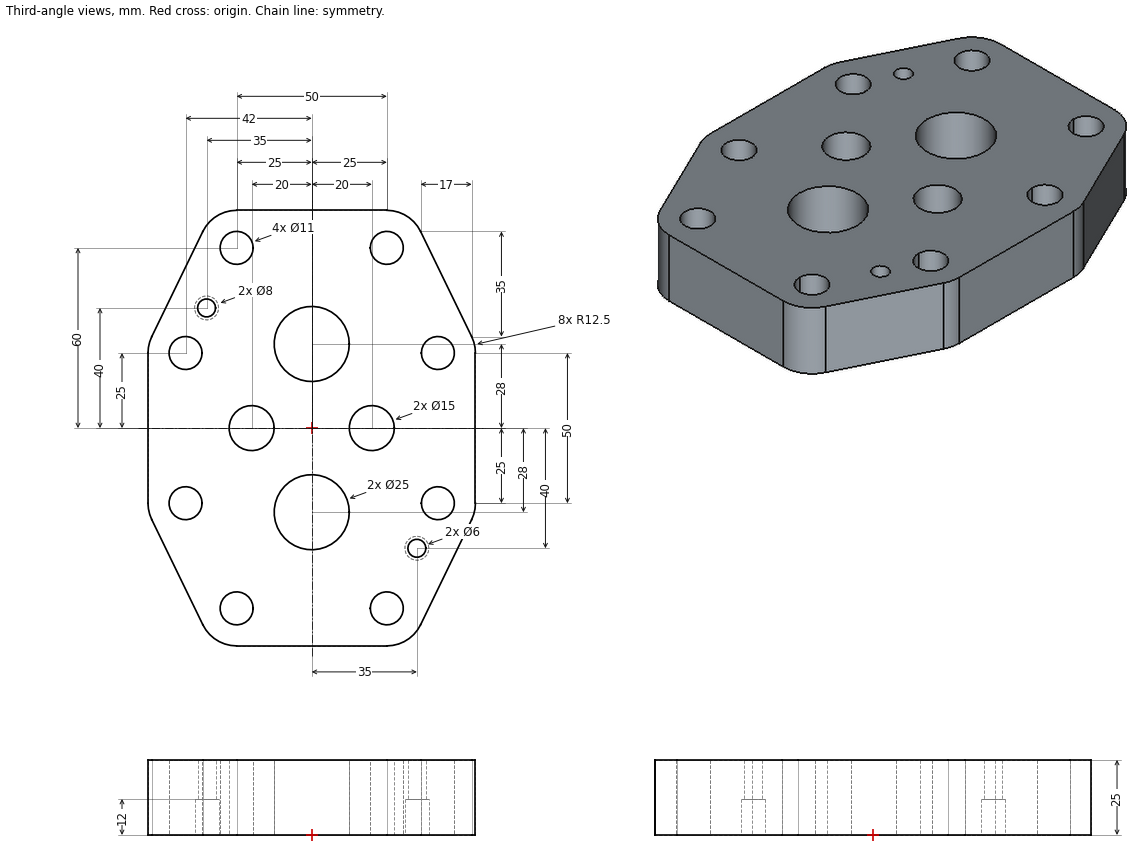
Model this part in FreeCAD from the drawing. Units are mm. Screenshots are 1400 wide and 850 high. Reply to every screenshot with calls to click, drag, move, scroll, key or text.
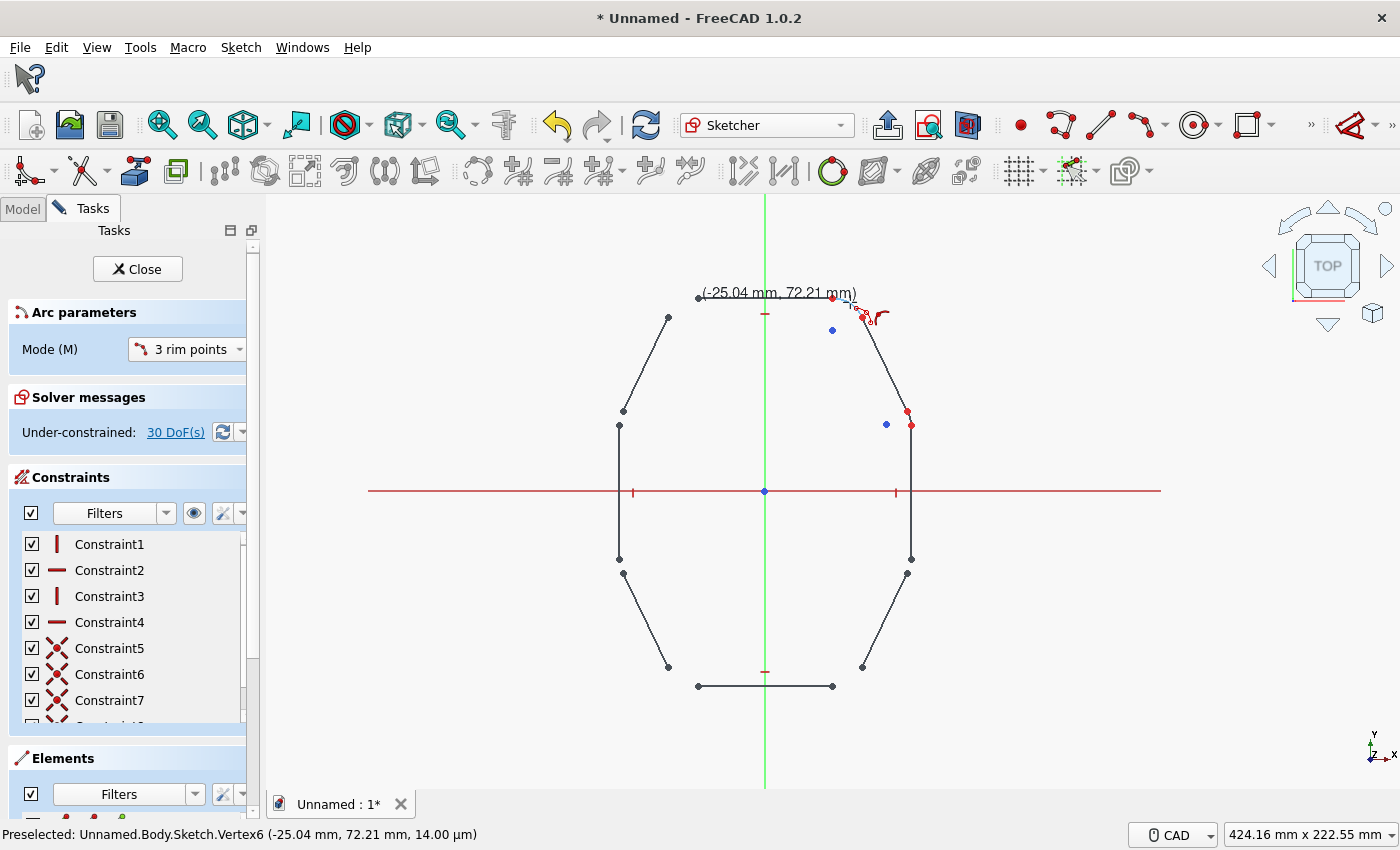
click(668, 317)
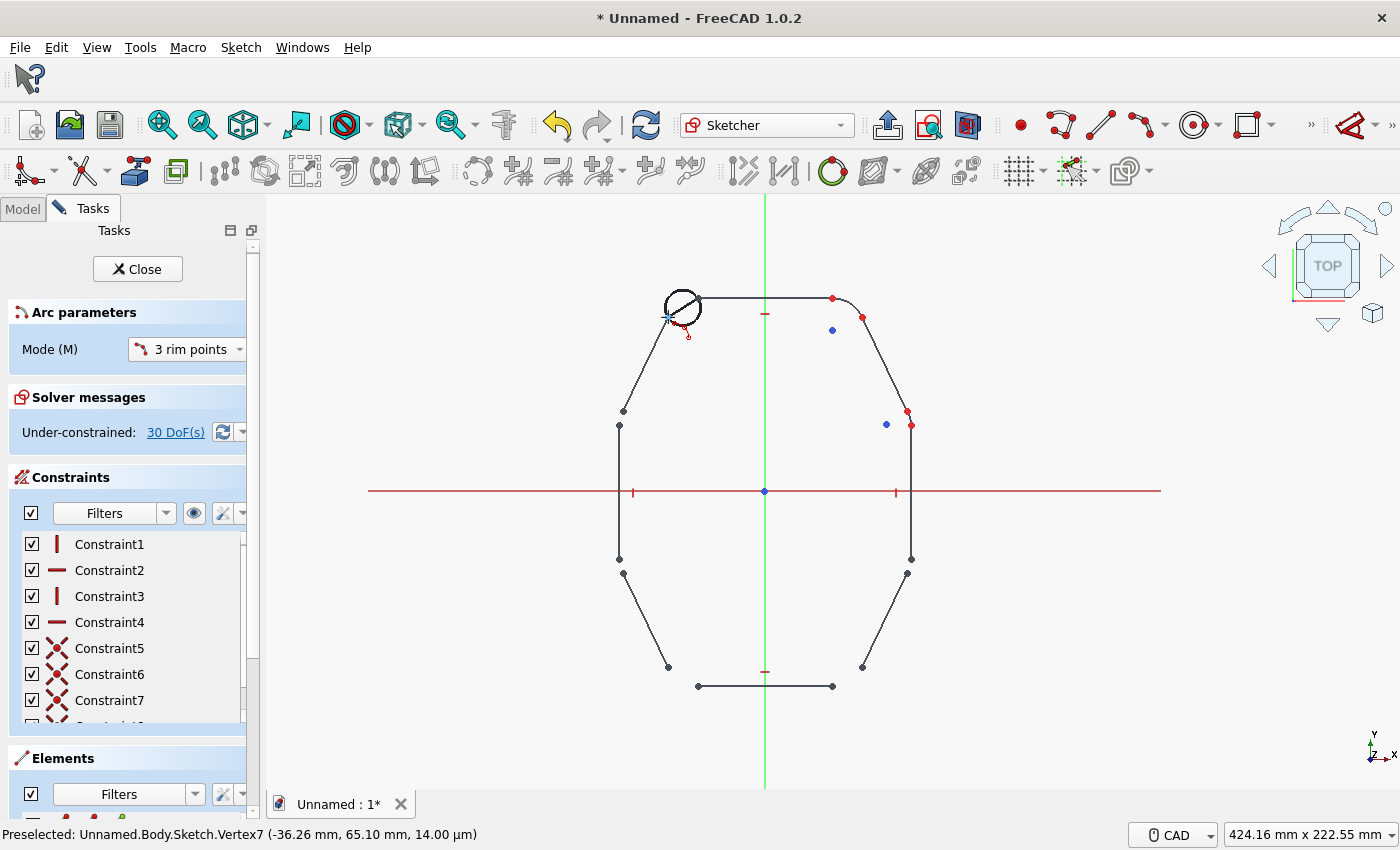
scroll(680, 303, up, 6)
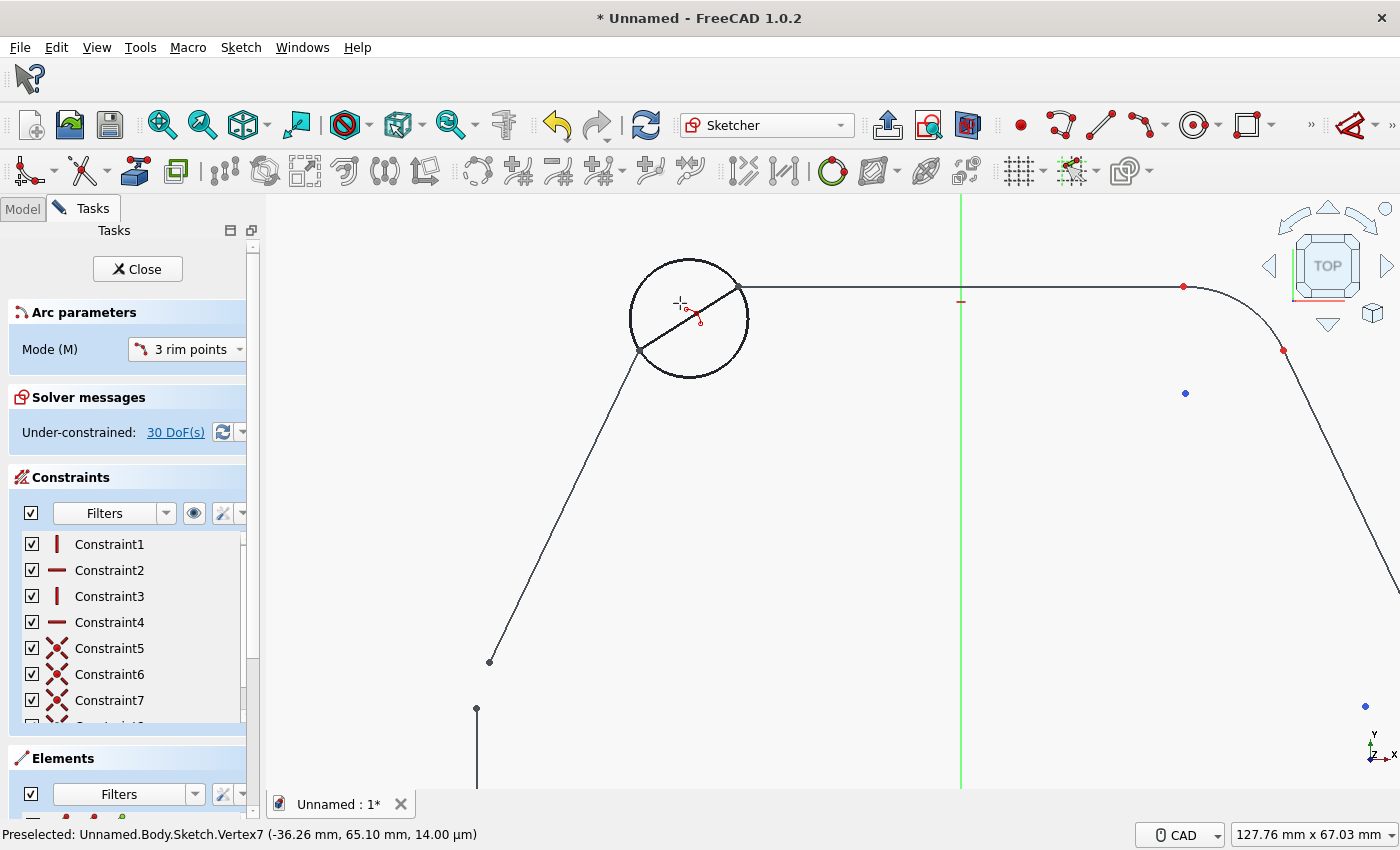
click(680, 301)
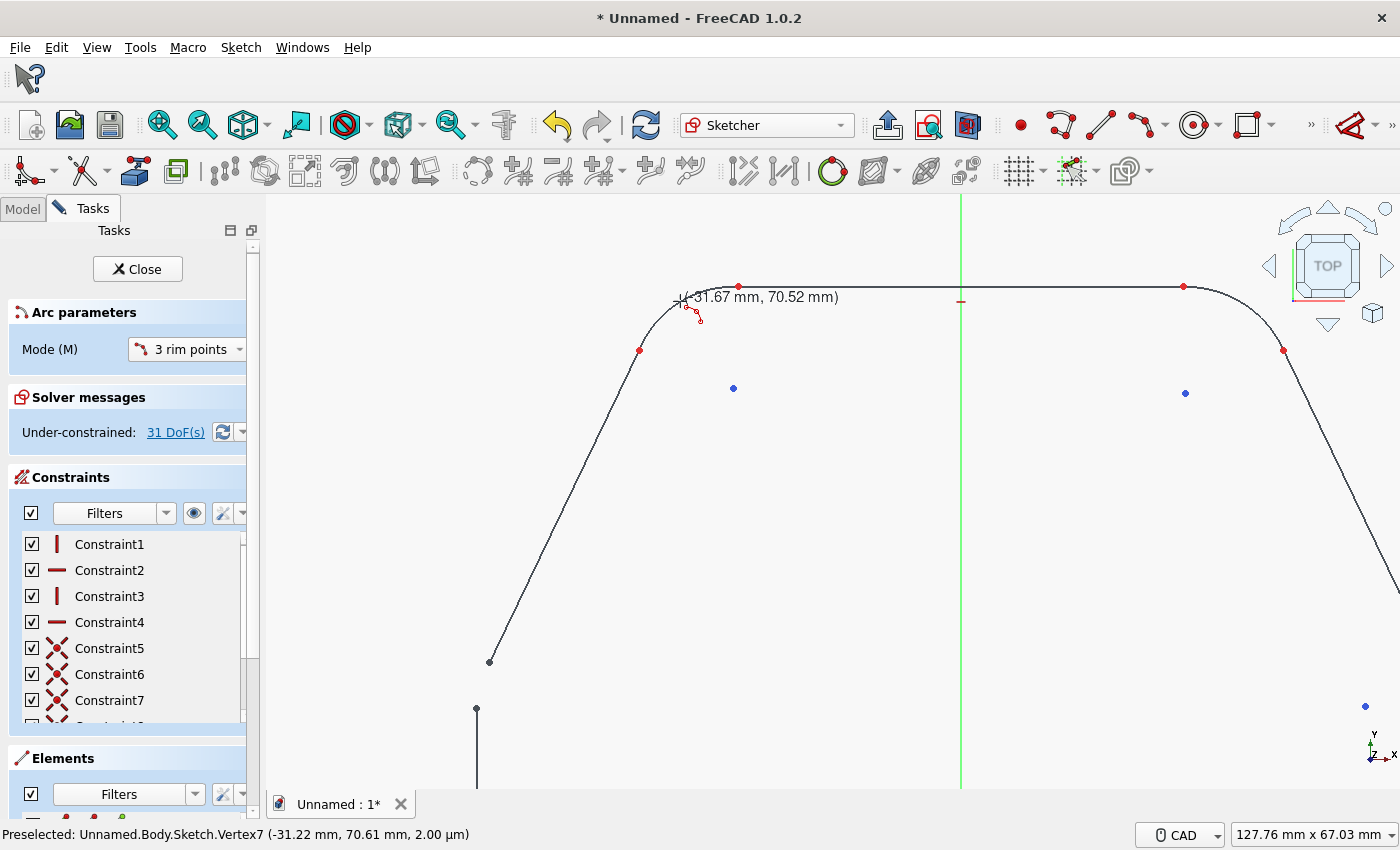
click(490, 662)
click(477, 709)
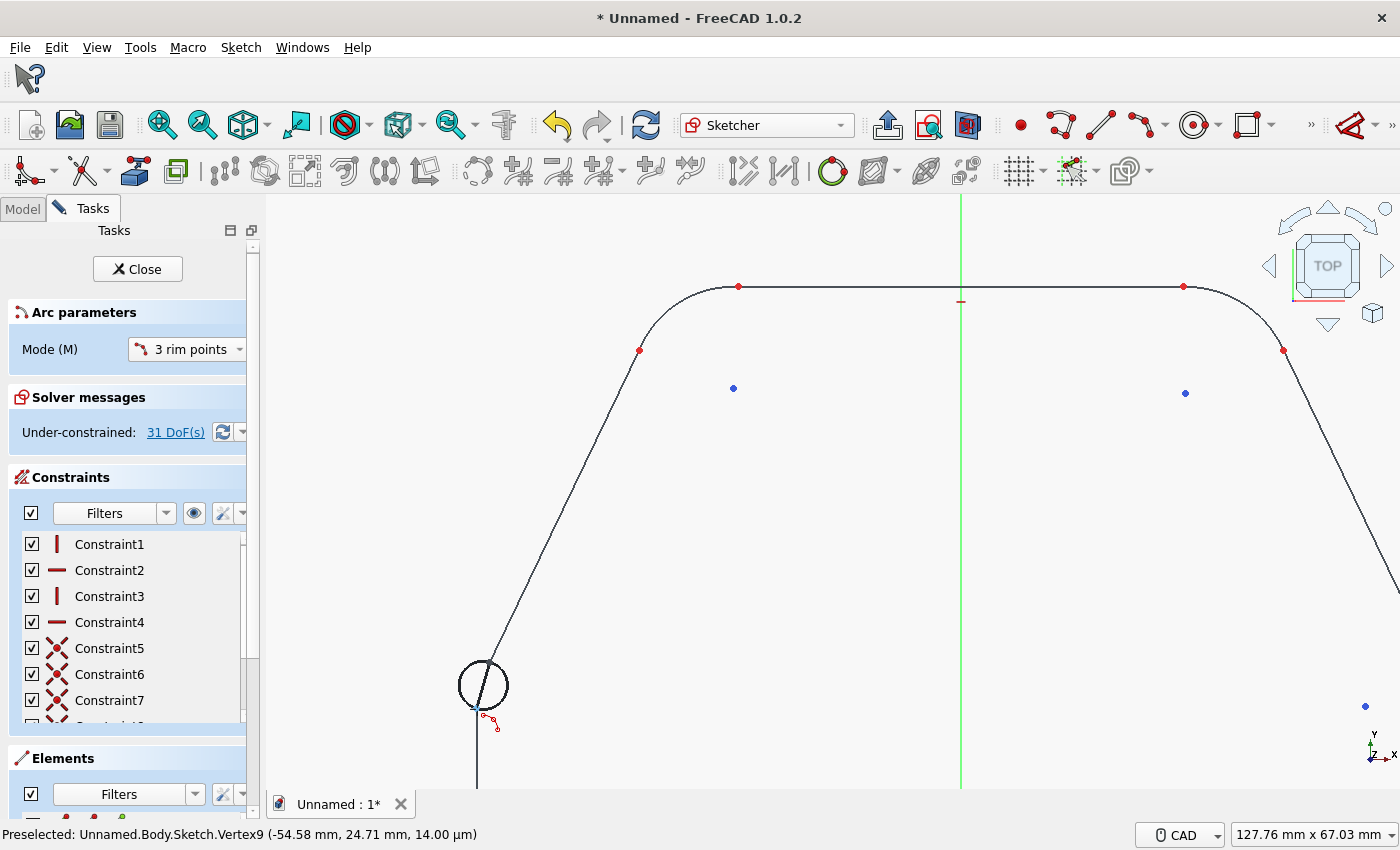
scroll(480, 681, up, 9)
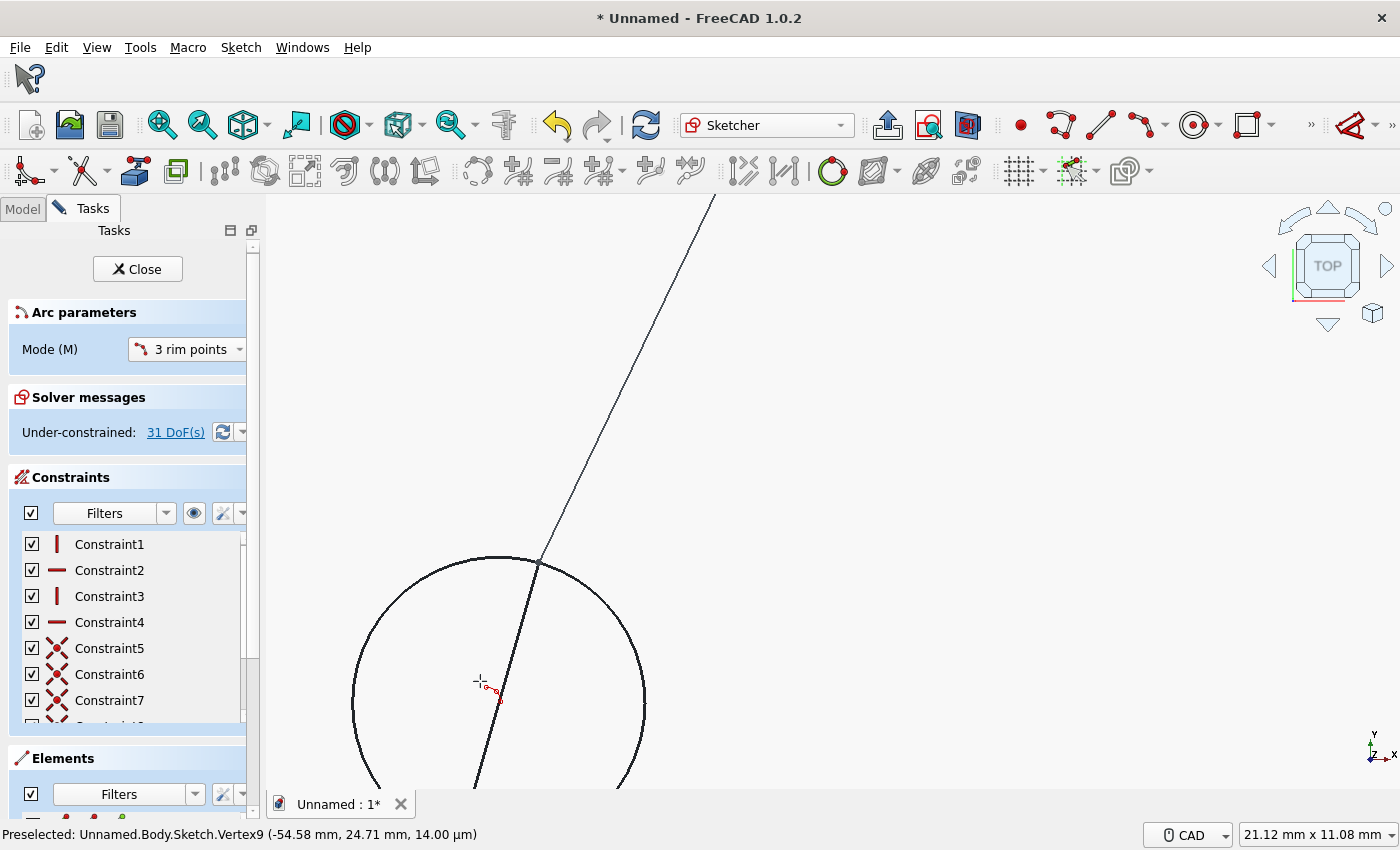
click(480, 678)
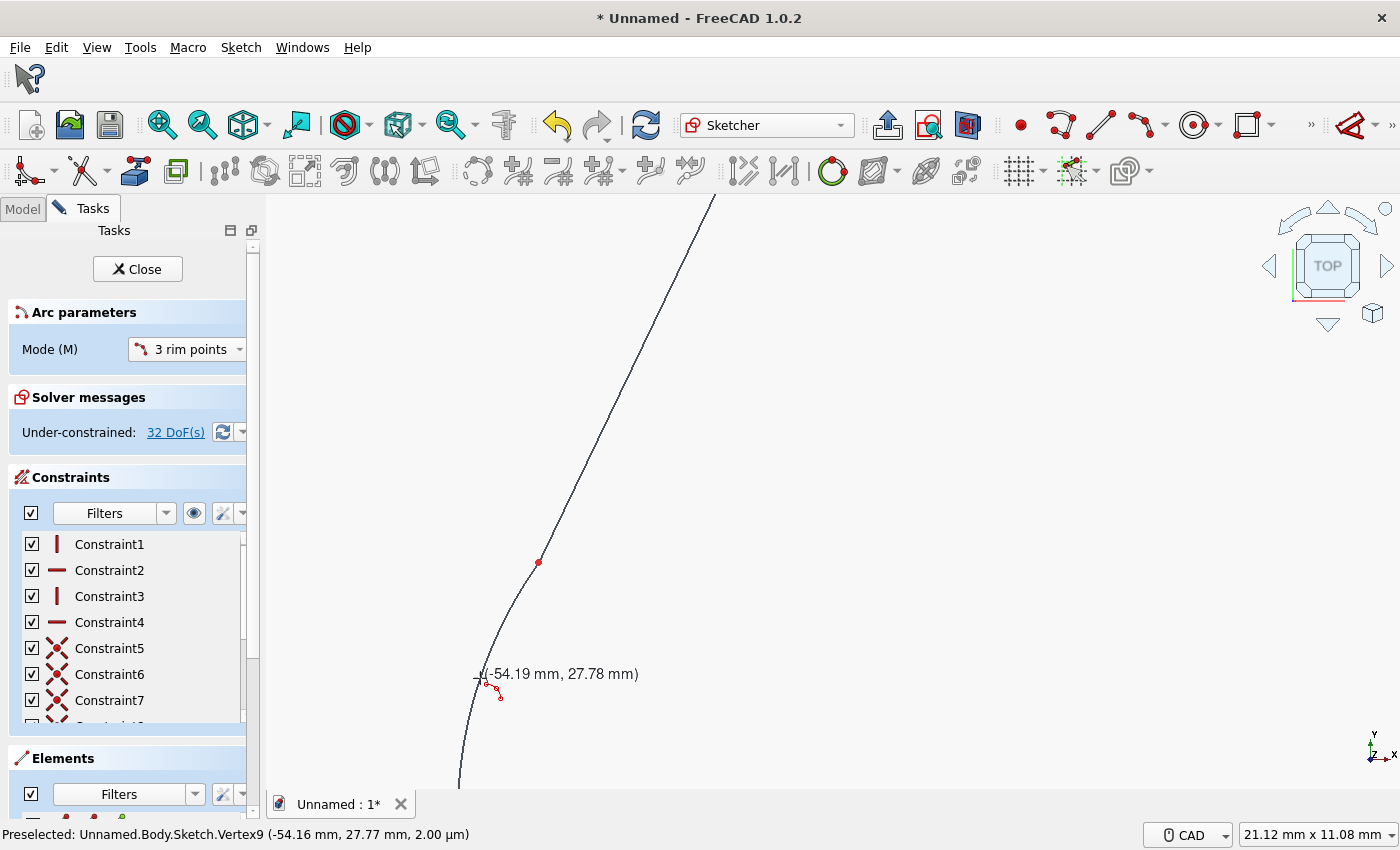
scroll(627, 404, down, 15)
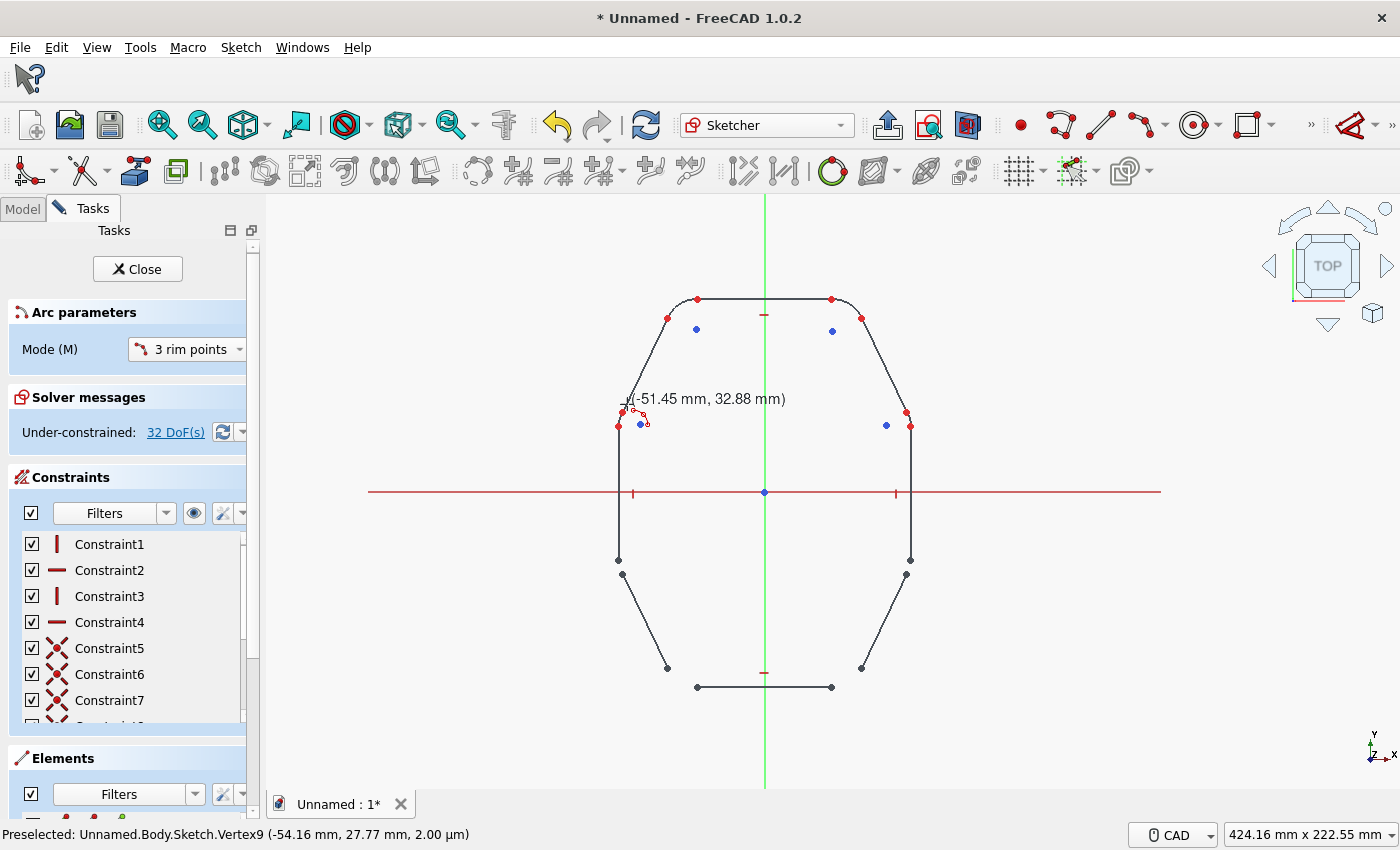
click(619, 560)
click(623, 574)